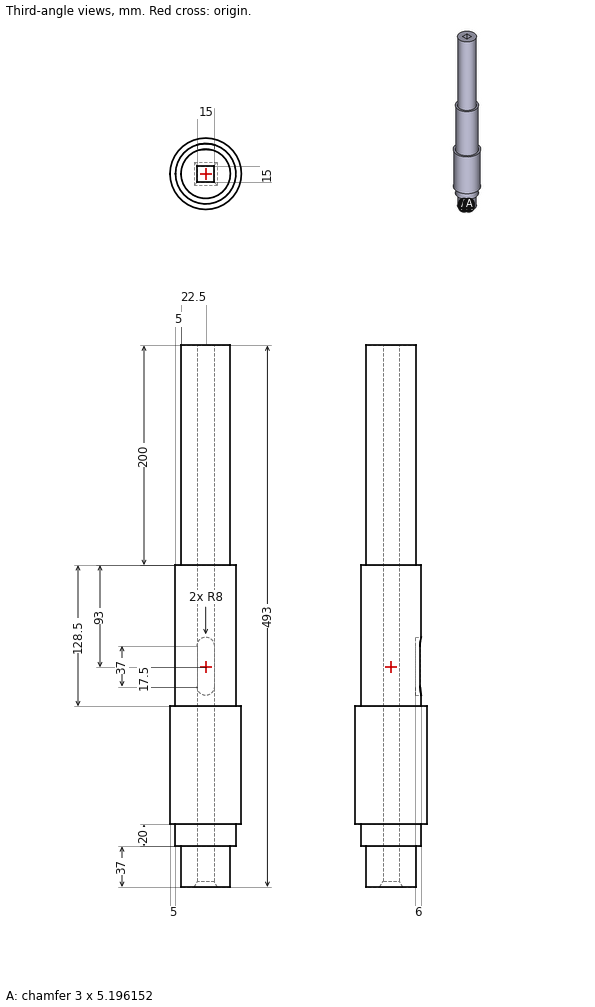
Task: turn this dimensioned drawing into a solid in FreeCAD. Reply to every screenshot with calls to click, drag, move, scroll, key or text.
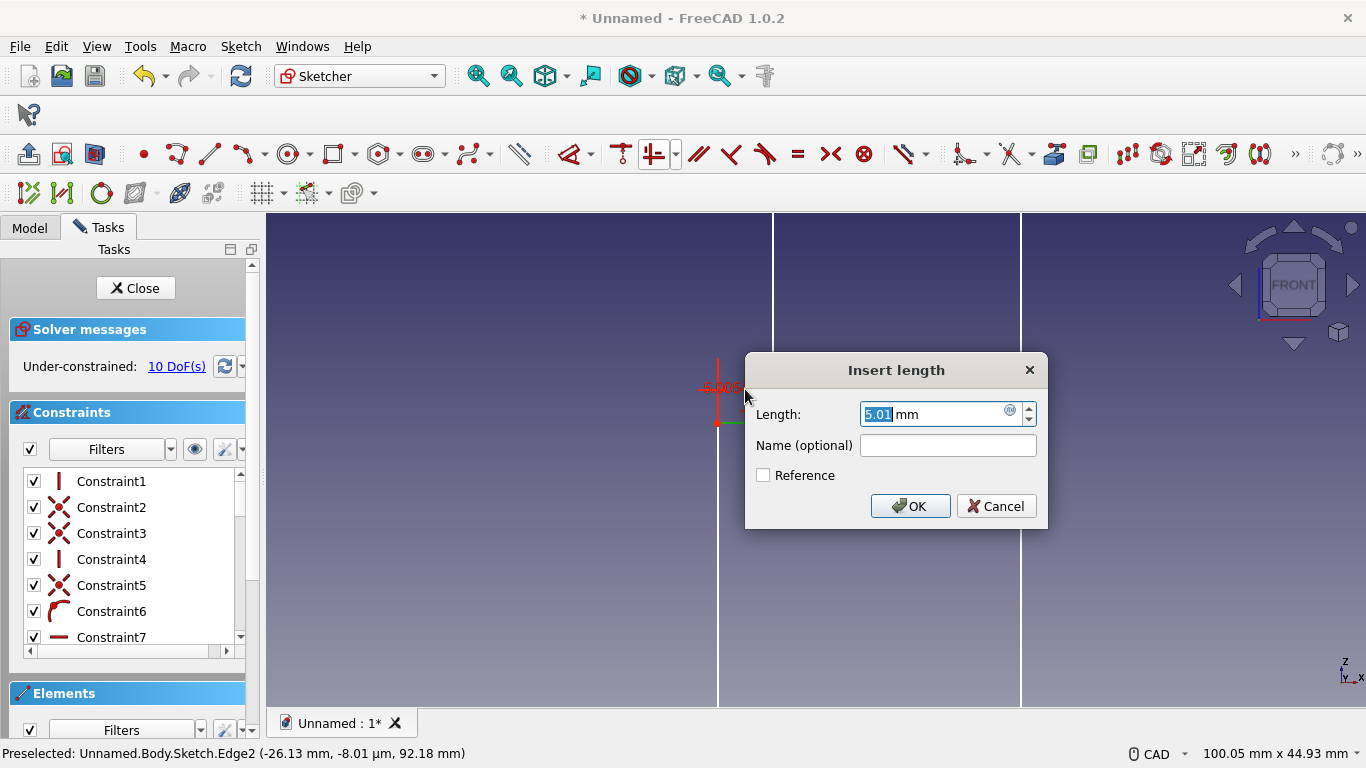
text(5)
key(Return)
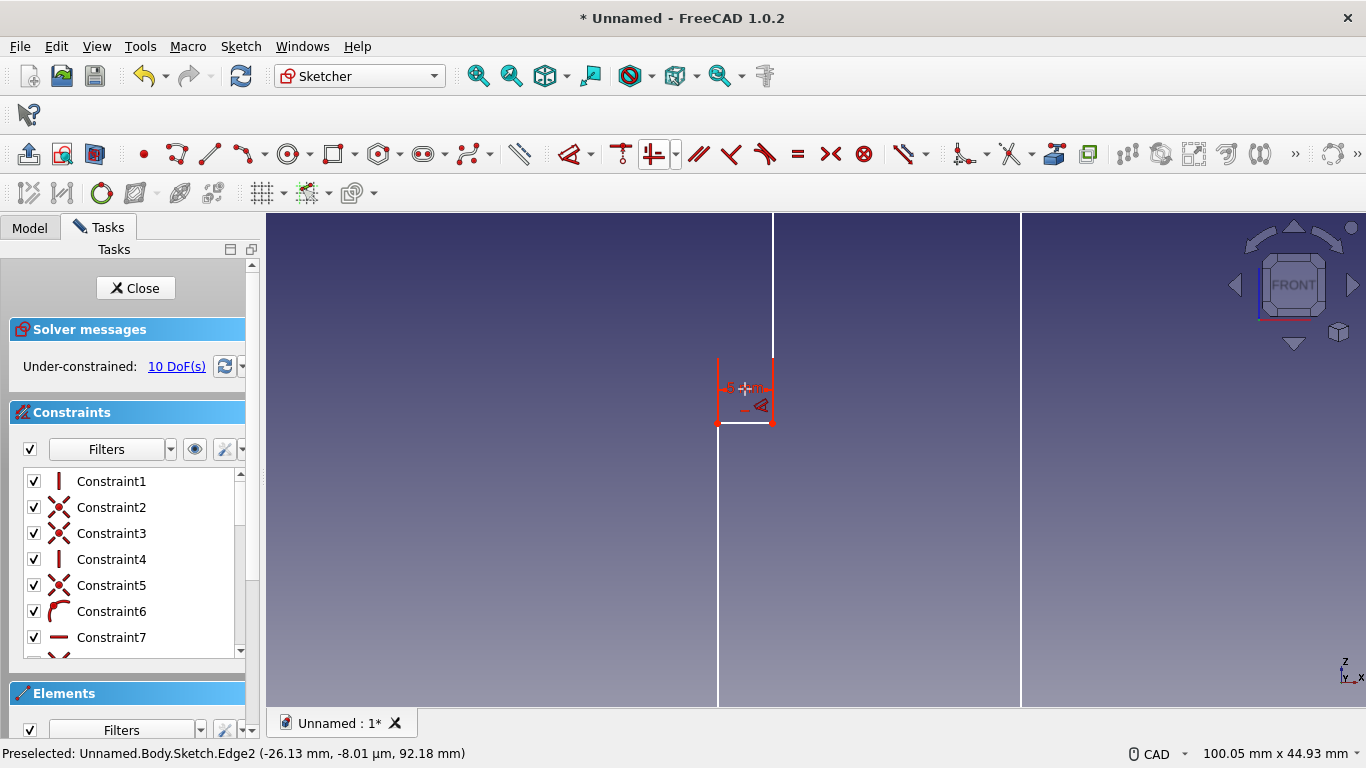
scroll(741, 430, down, 14)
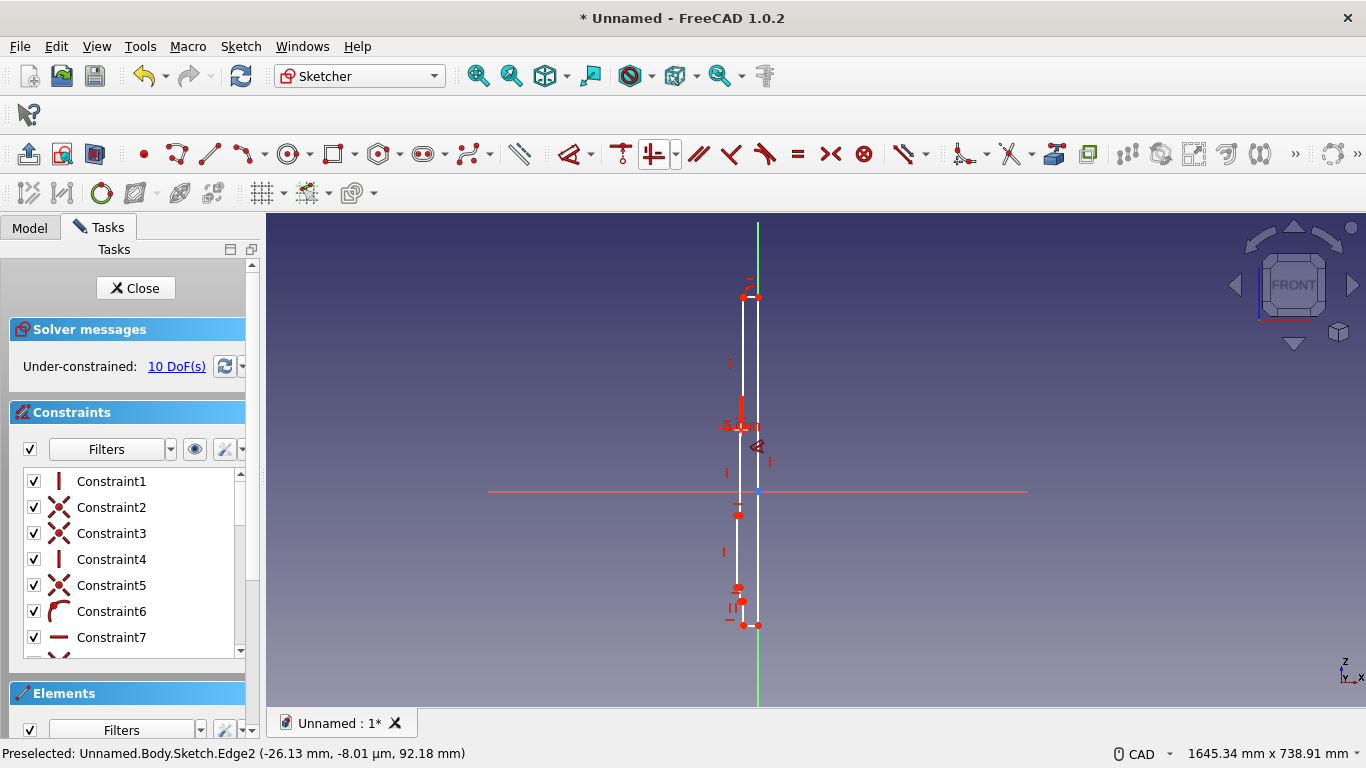
scroll(742, 602, up, 14)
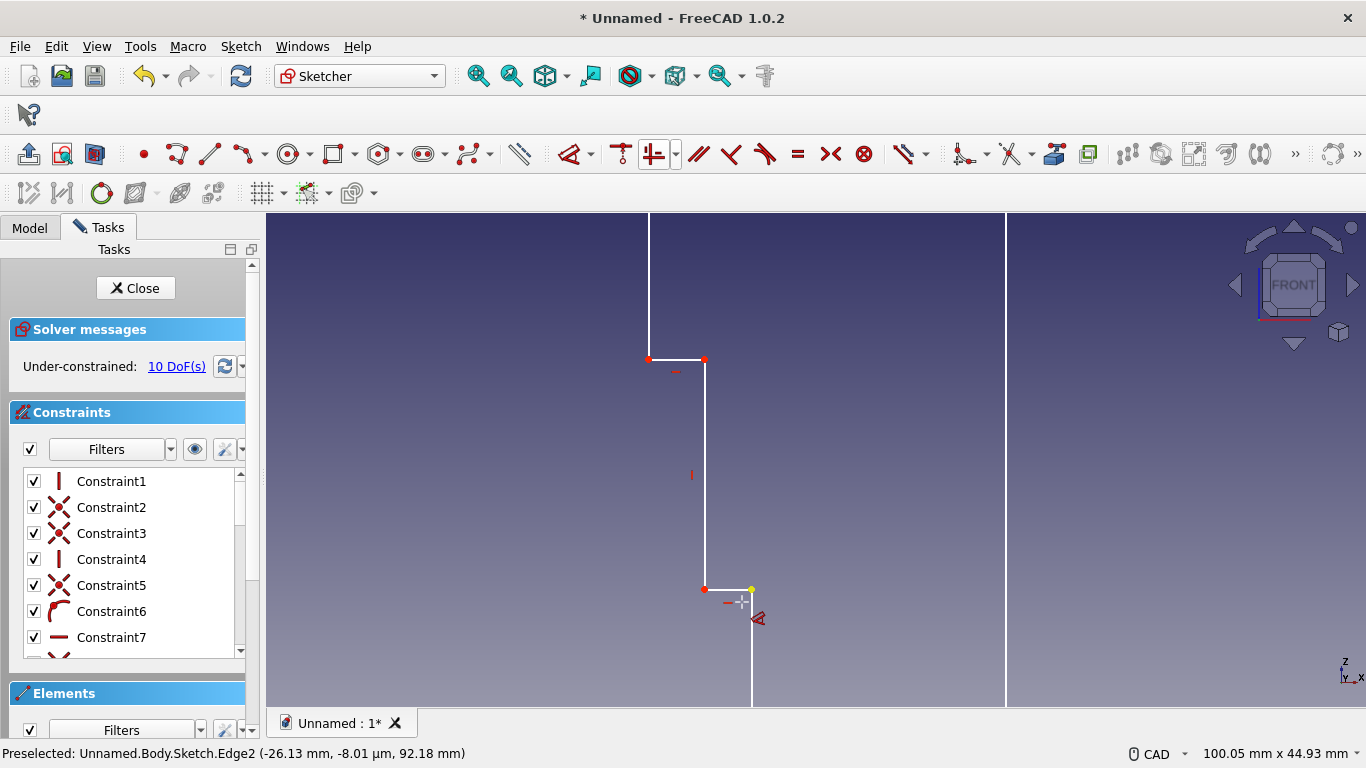
click(738, 590)
click(728, 624)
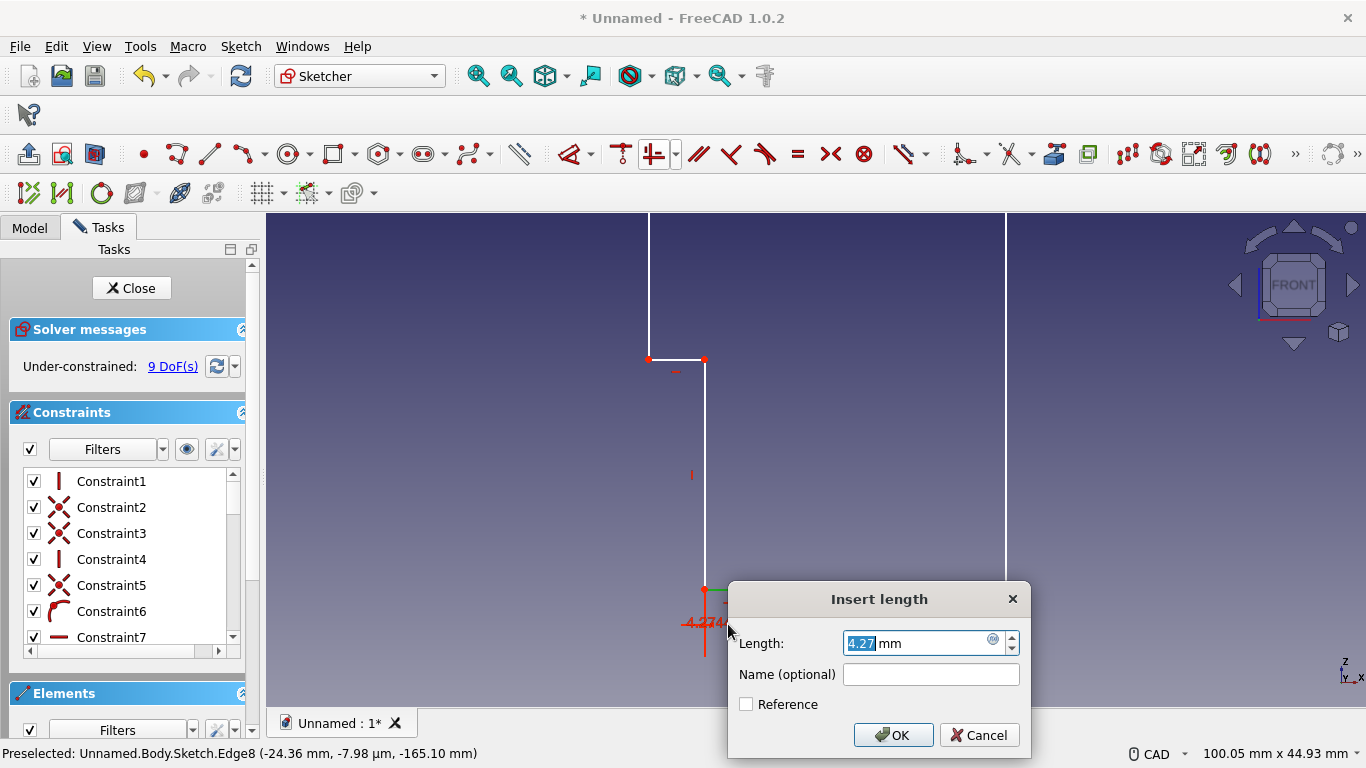
text(5)
key(Return)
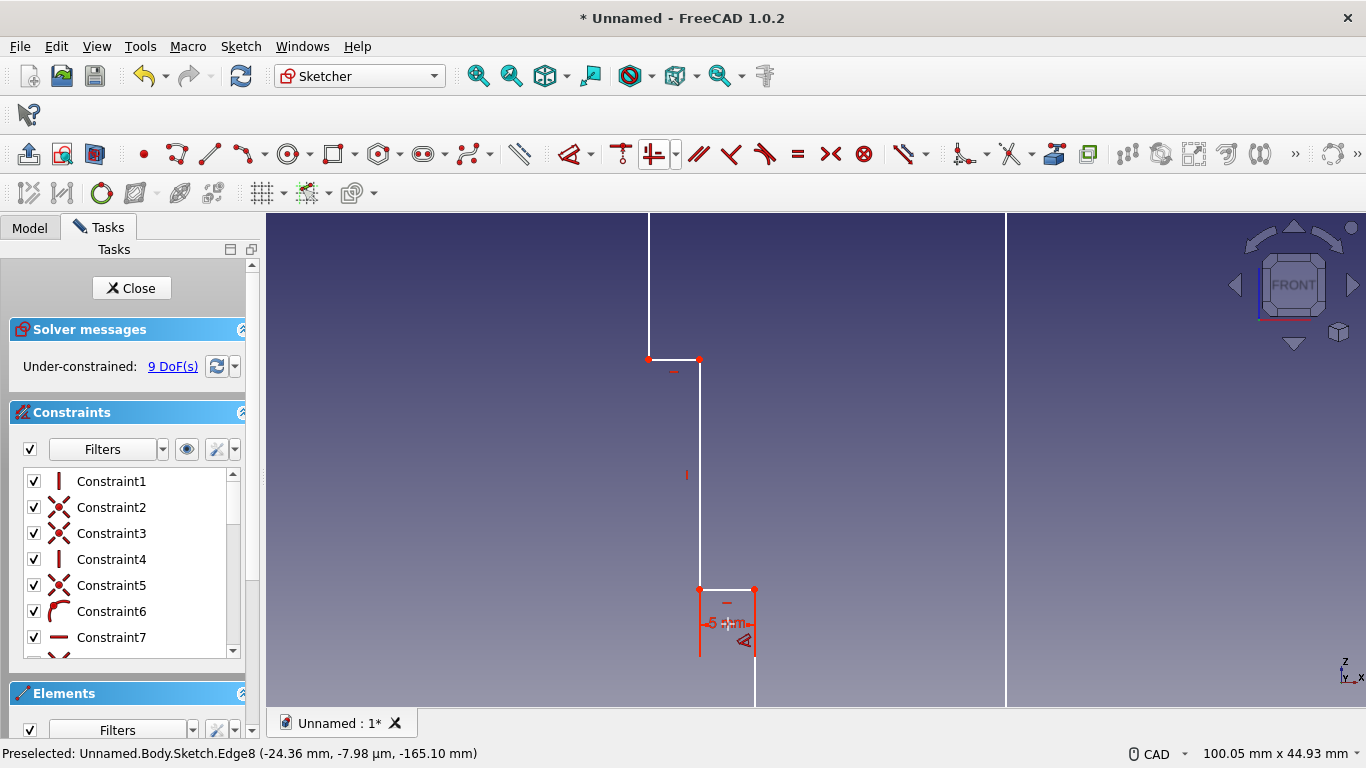
click(685, 360)
click(674, 394)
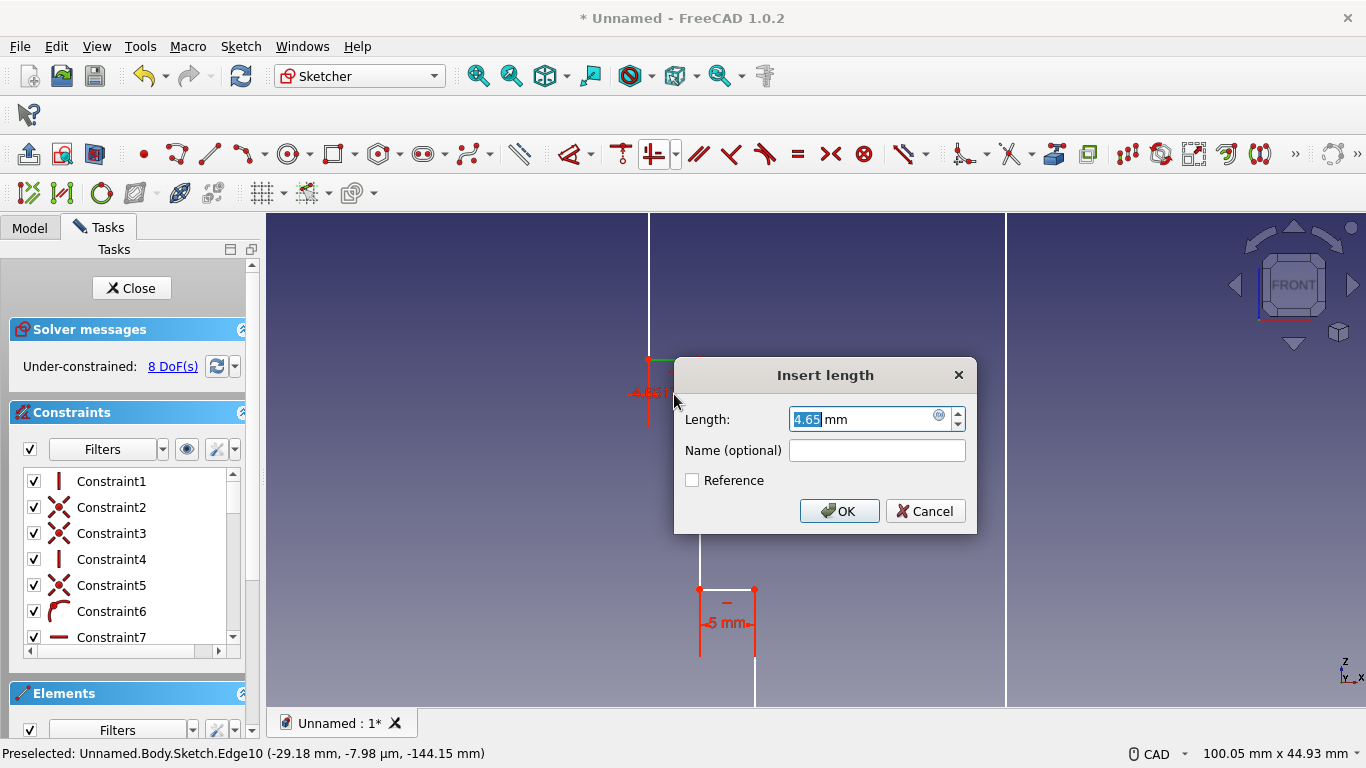
text(5)
key(Return)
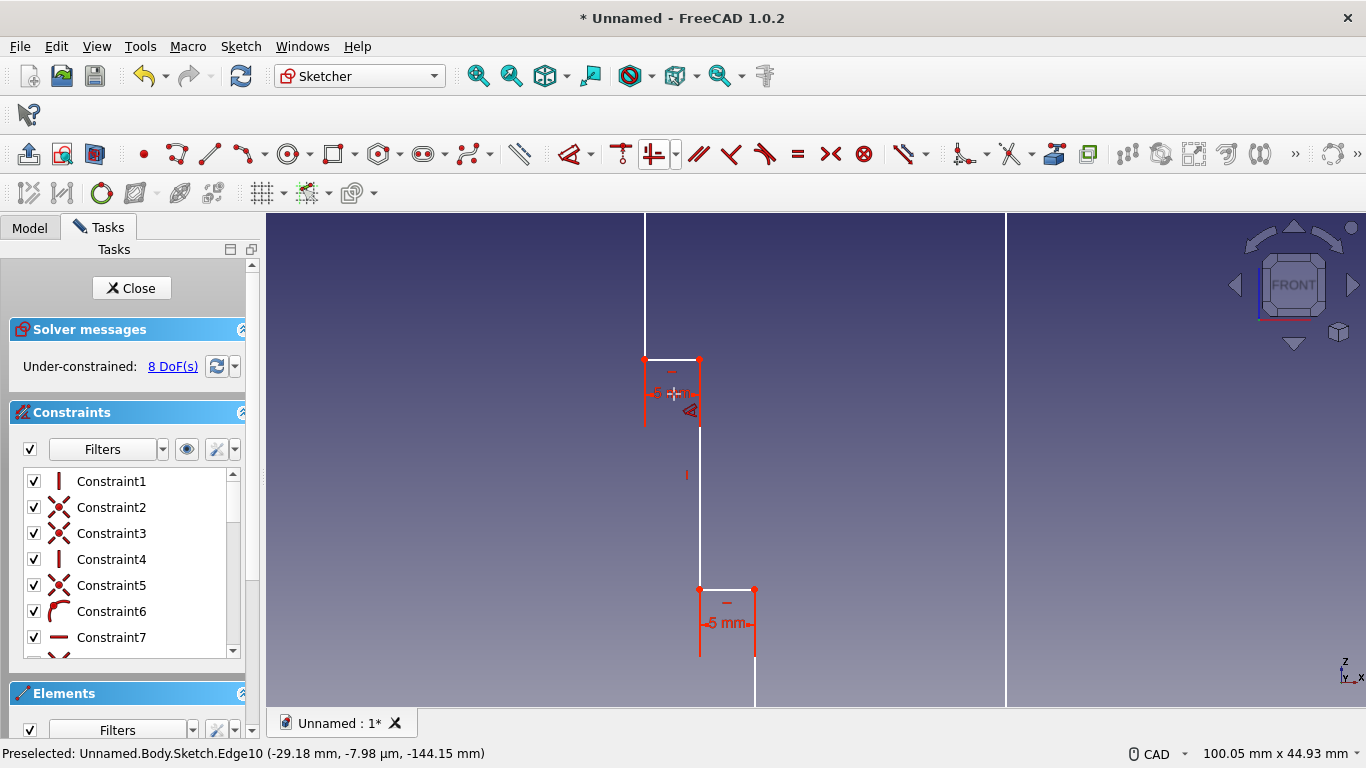
scroll(742, 602, down, 14)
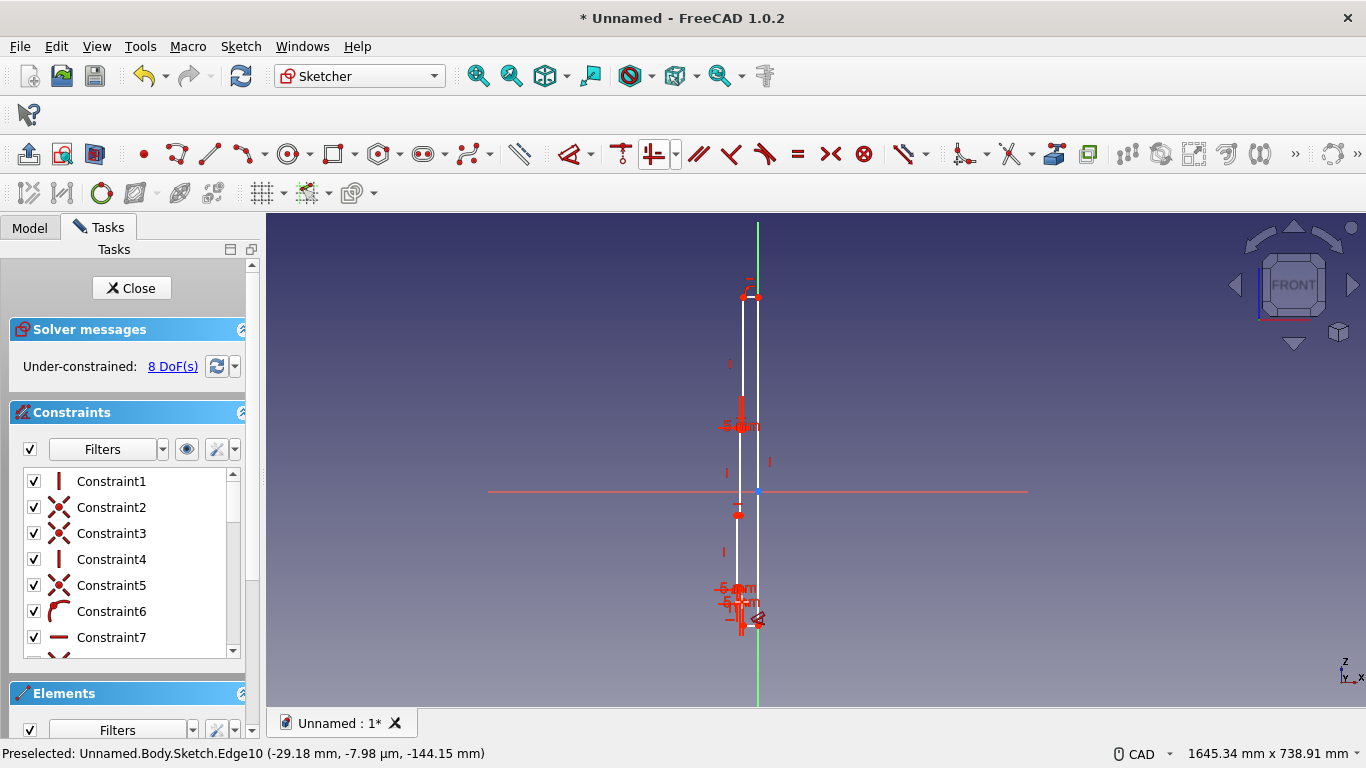
scroll(738, 515, up, 13)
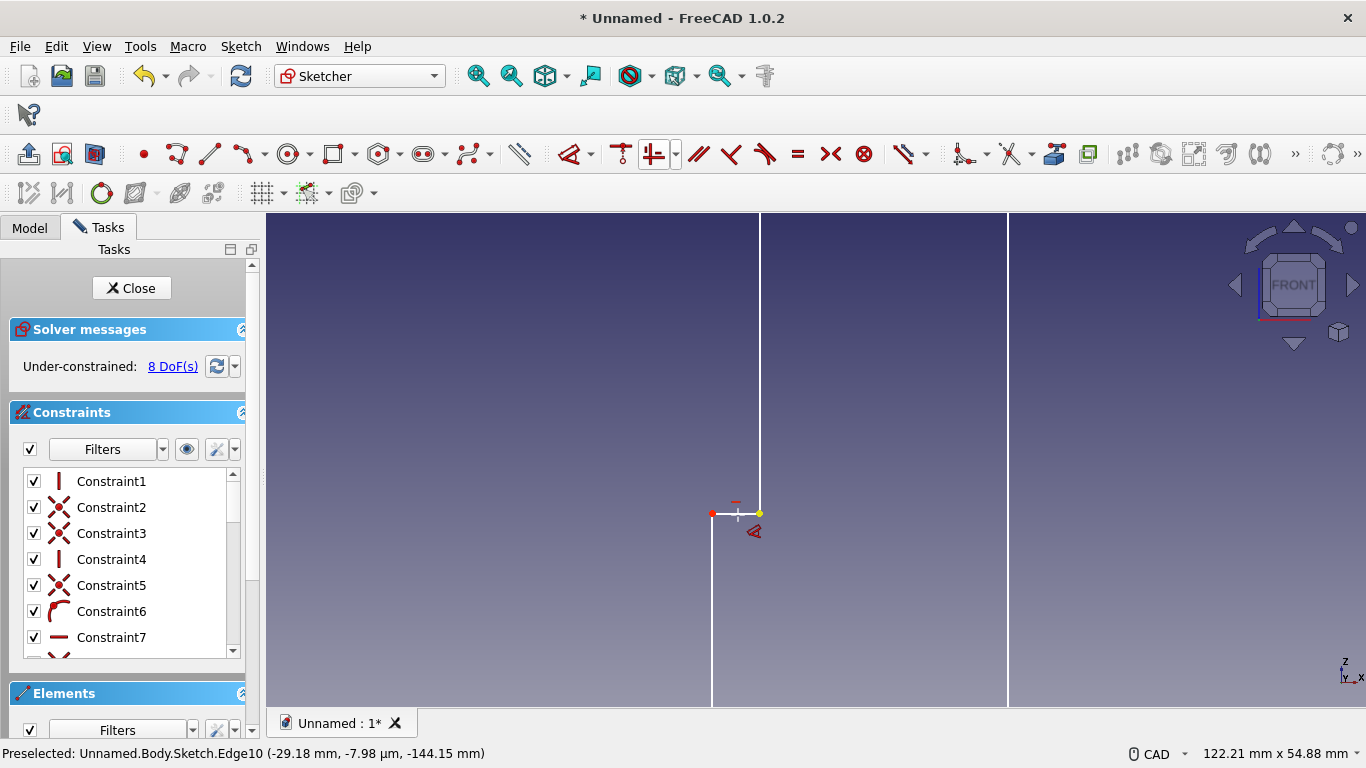
click(727, 514)
click(736, 548)